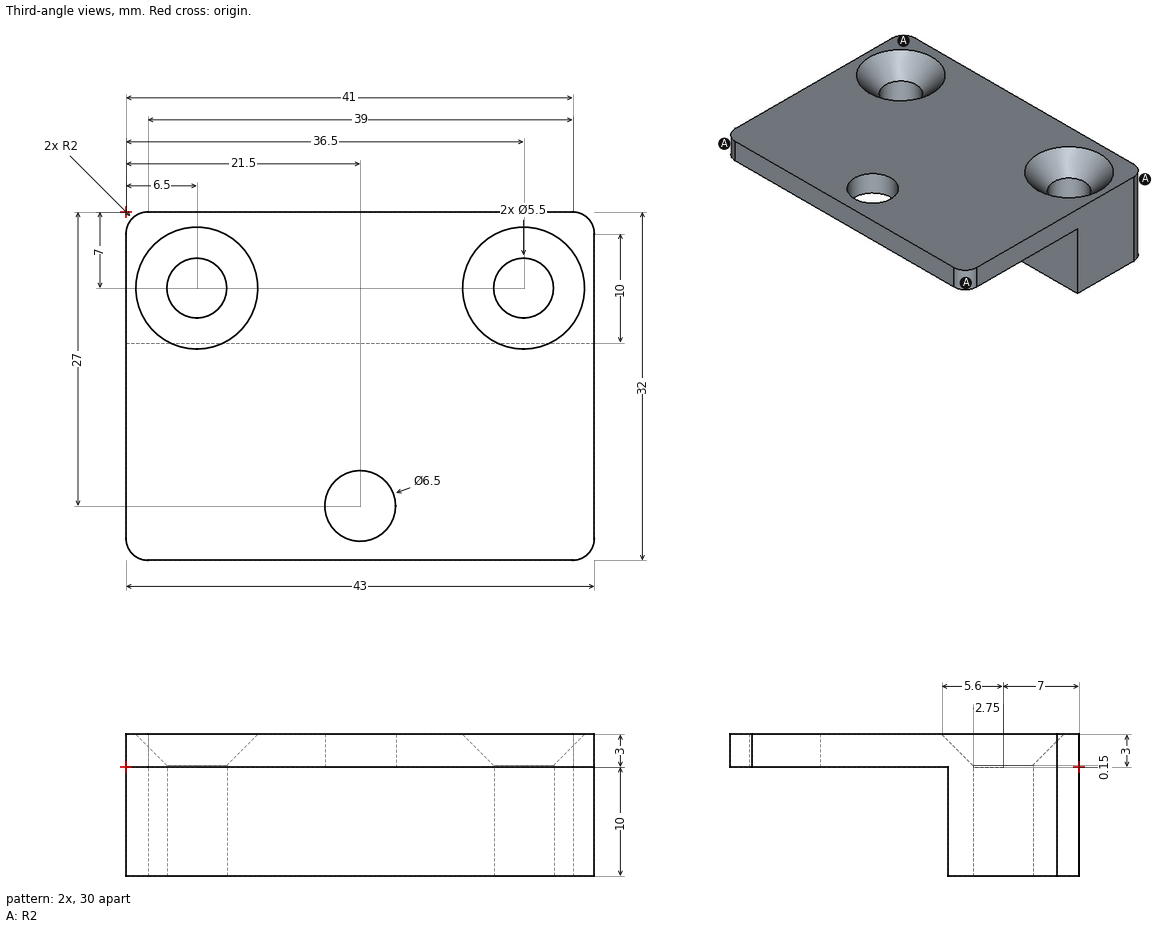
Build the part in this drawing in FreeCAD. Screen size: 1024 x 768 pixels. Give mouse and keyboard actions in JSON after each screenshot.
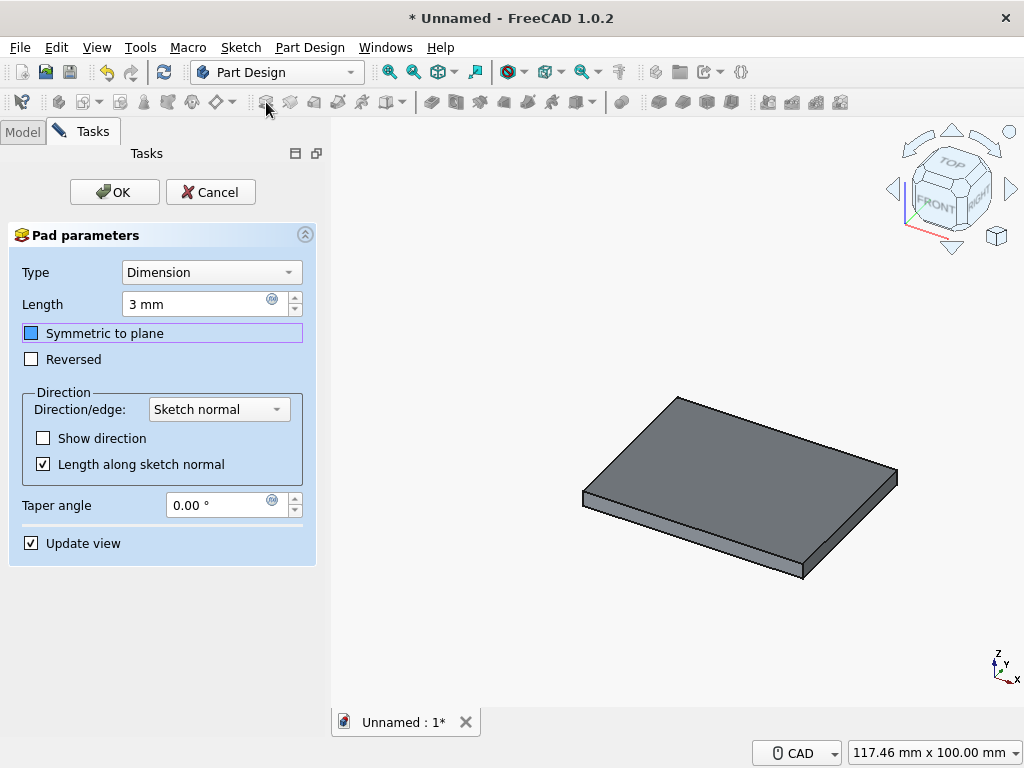
{"action": "left_click", "coordinate": [115, 192]}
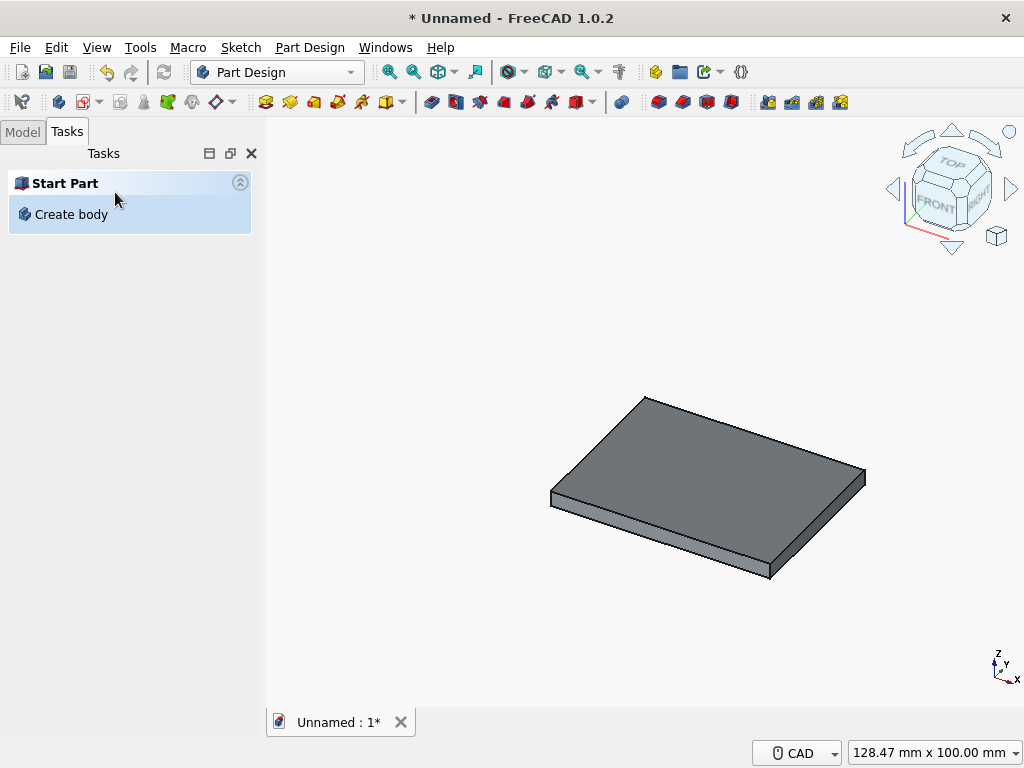
{"action": "key", "text": "v f"}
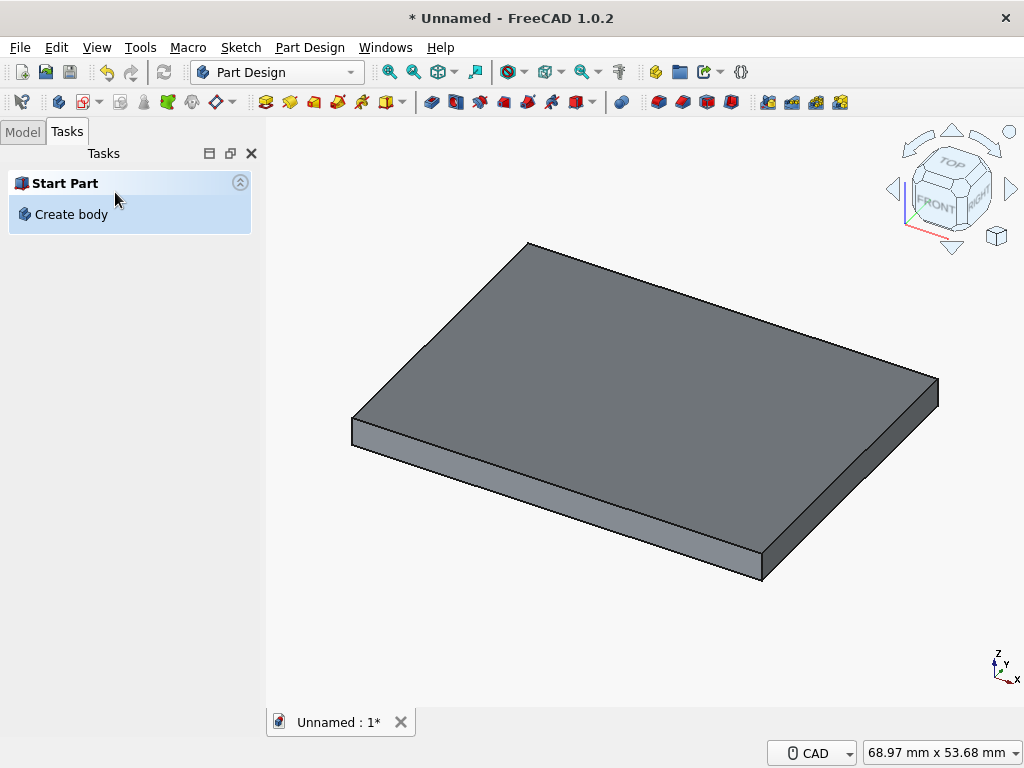
{"action": "left_click", "coordinate": [23, 131]}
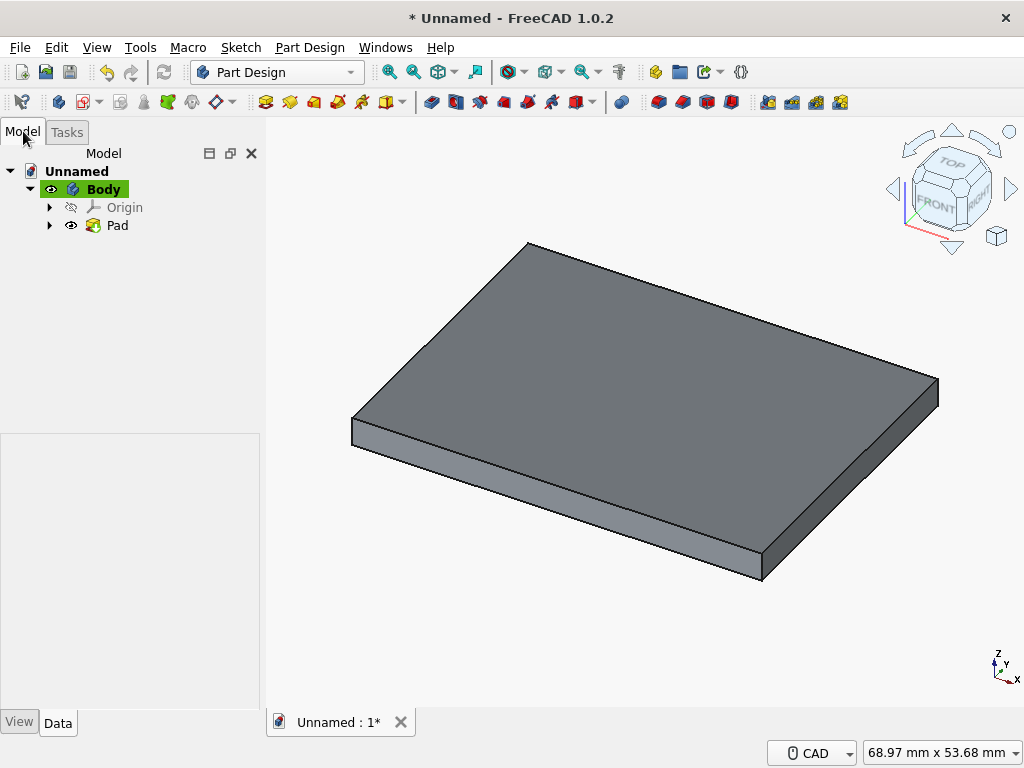
{"action": "left_click", "coordinate": [50, 207]}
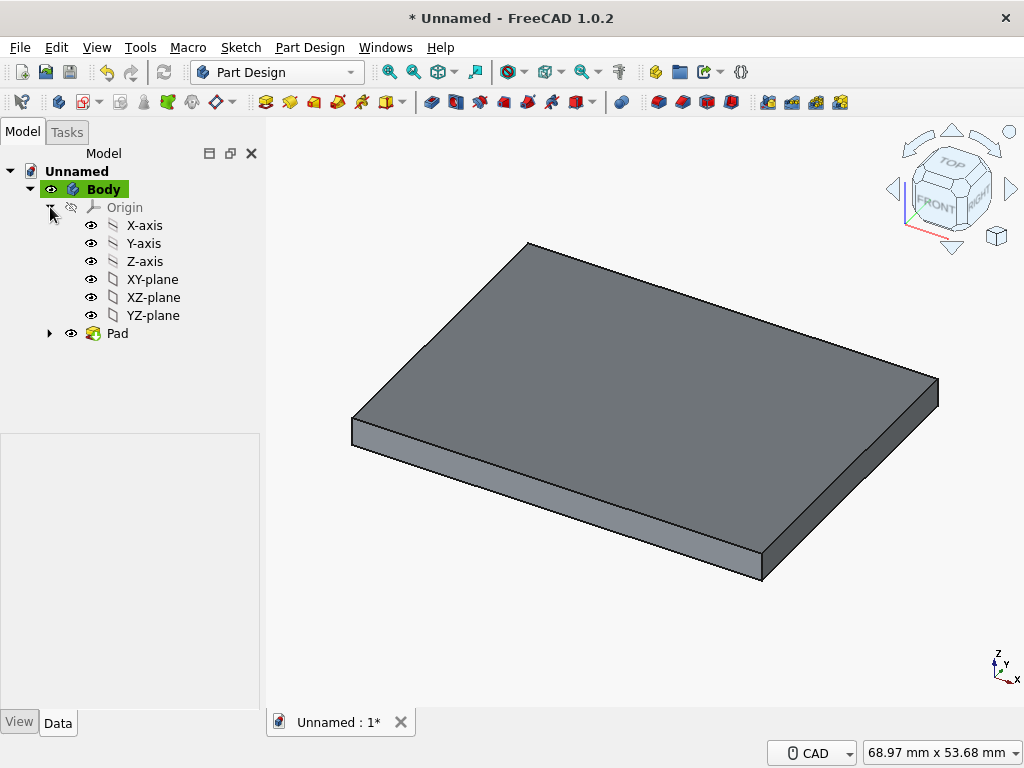
{"action": "left_click", "coordinate": [136, 315]}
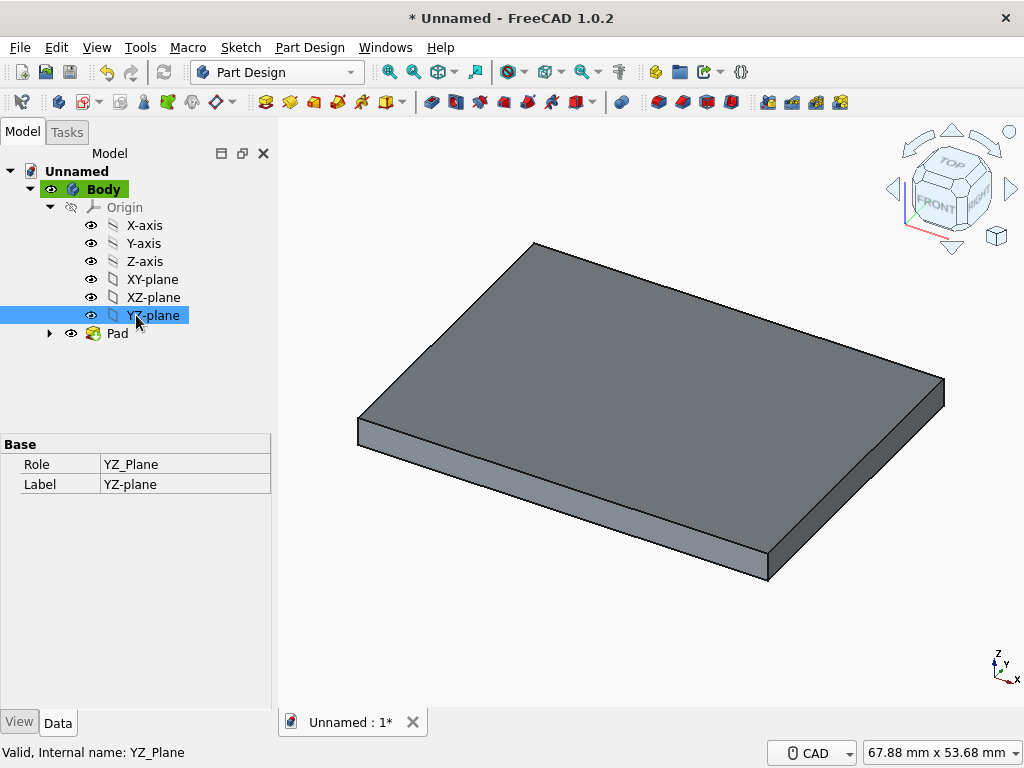
{"action": "left_click", "coordinate": [216, 102]}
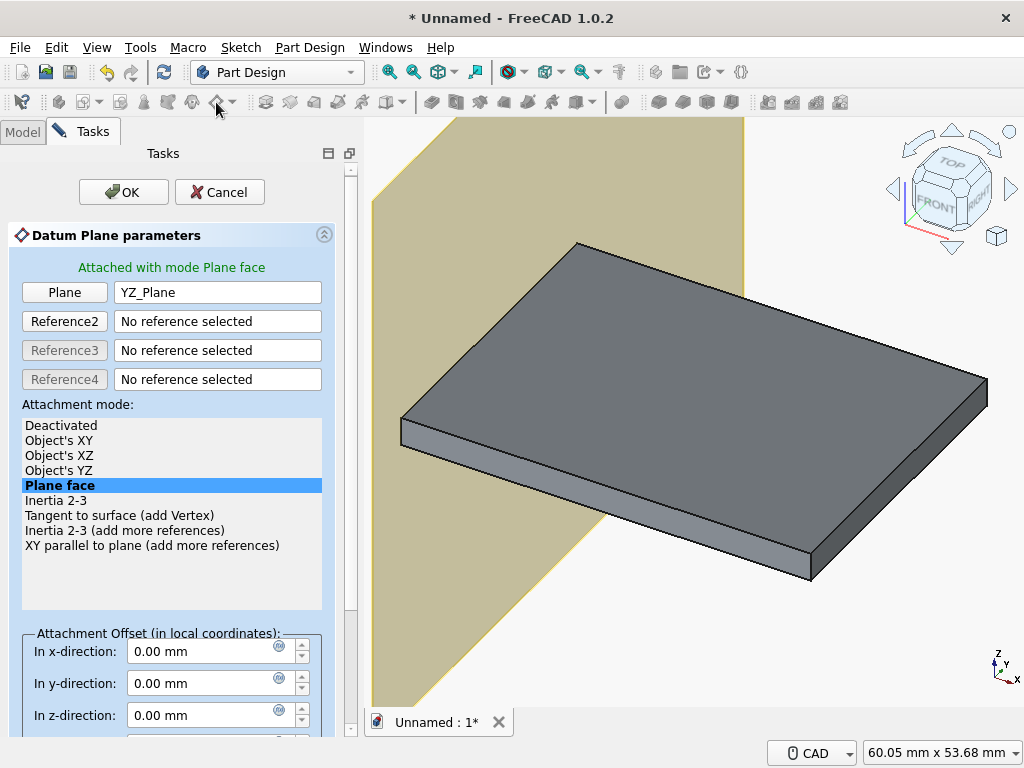
{"action": "triple_click", "coordinate": [210, 715]}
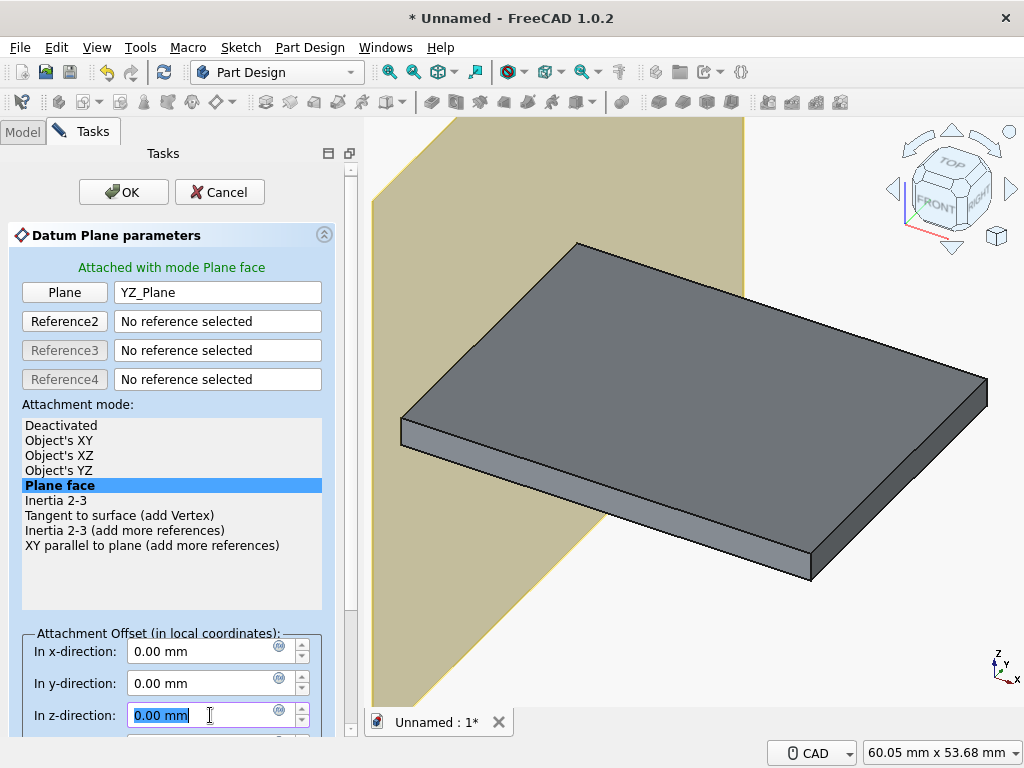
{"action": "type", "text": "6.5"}
{"action": "key", "text": "Tab"}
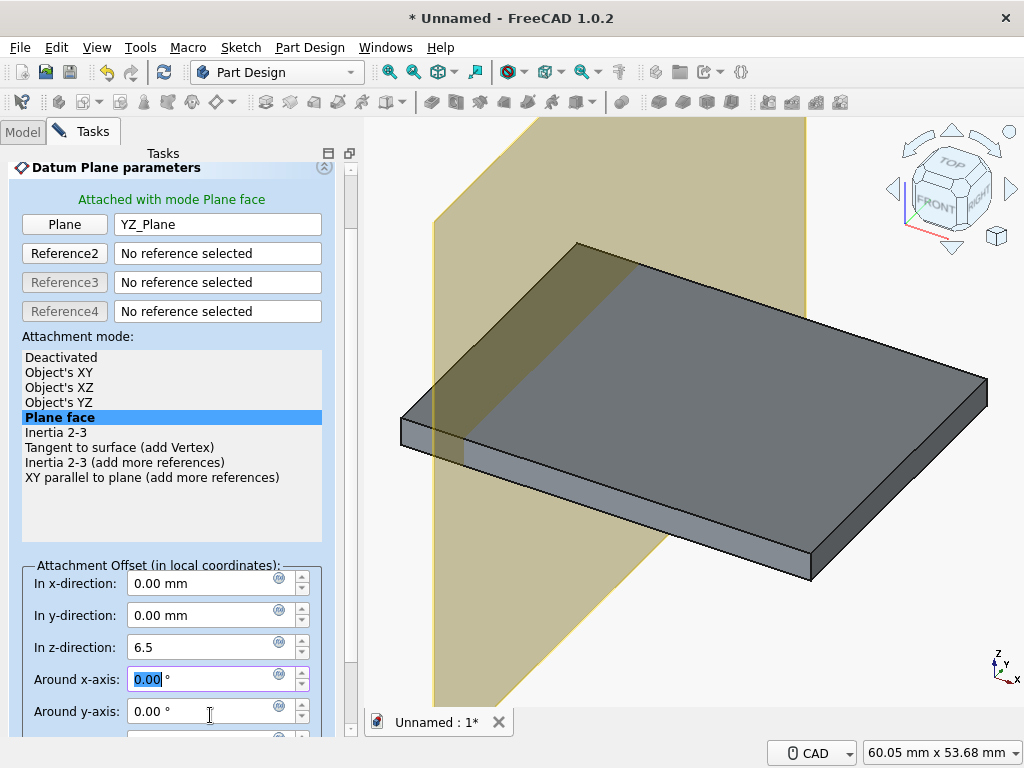
{"action": "scroll", "coordinate": [351, 450], "scroll_direction": "up", "scroll_amount": 2}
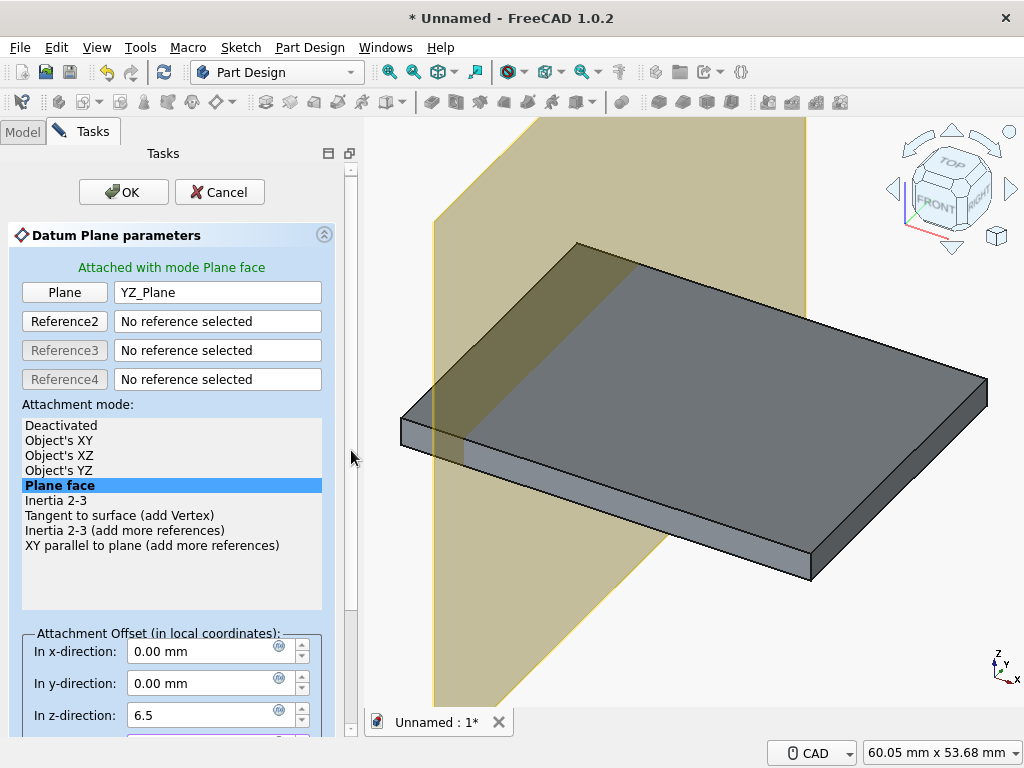
{"action": "left_click", "coordinate": [124, 192]}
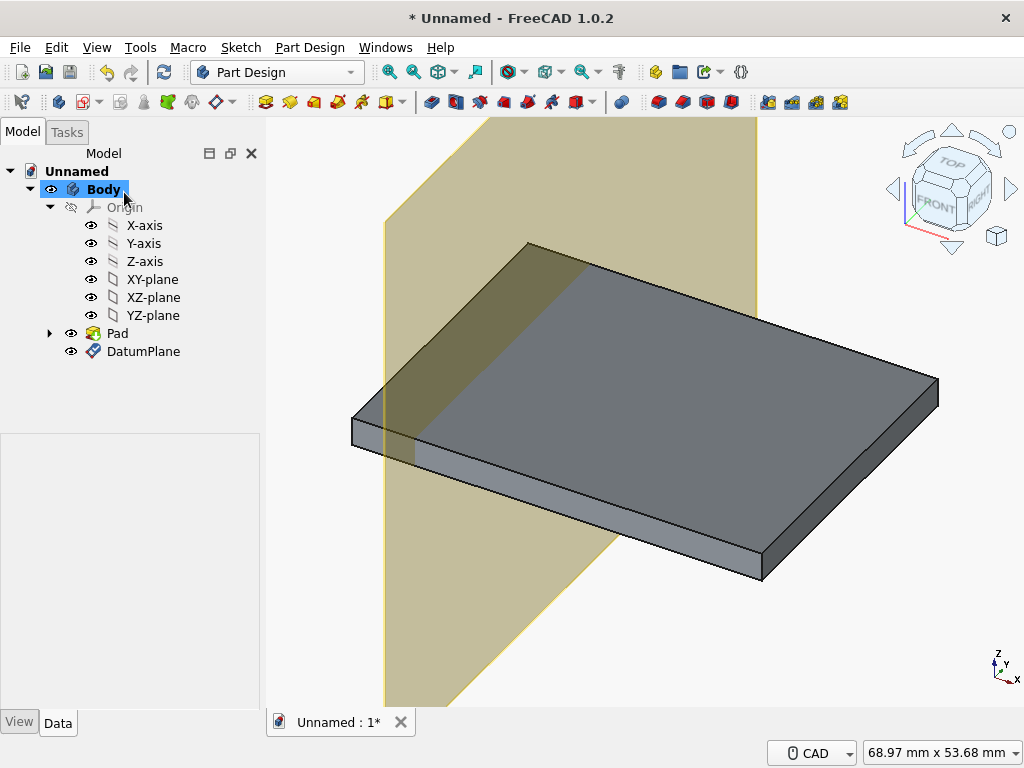
{"action": "left_click", "coordinate": [116, 351]}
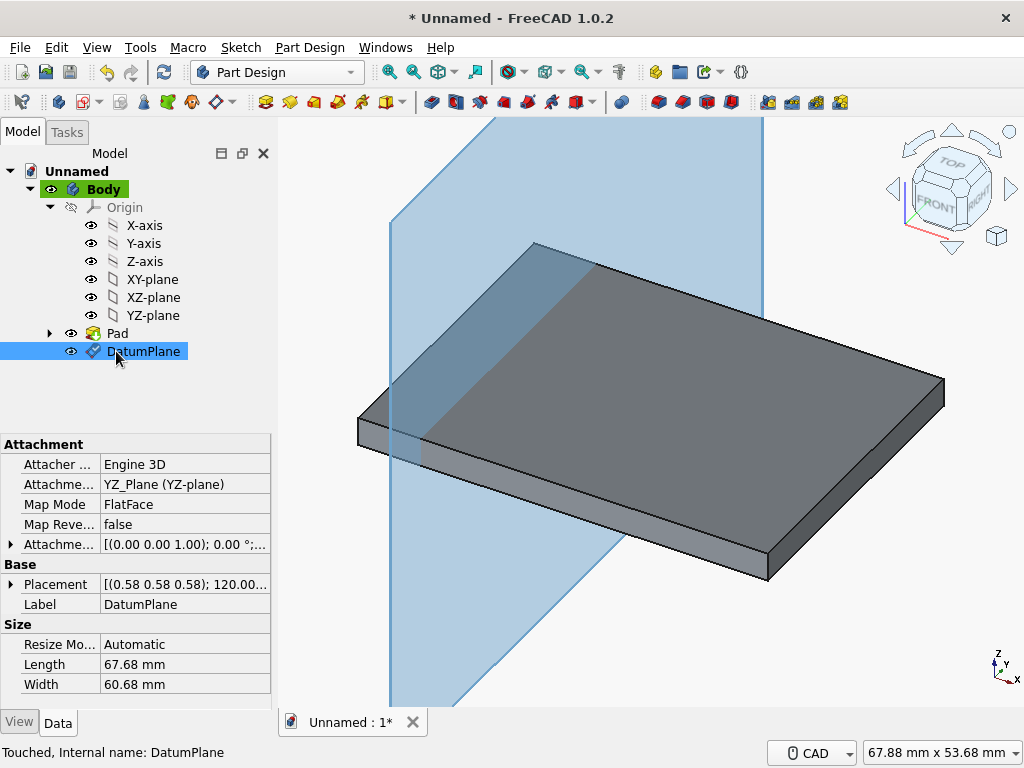
{"action": "left_click", "coordinate": [84, 102]}